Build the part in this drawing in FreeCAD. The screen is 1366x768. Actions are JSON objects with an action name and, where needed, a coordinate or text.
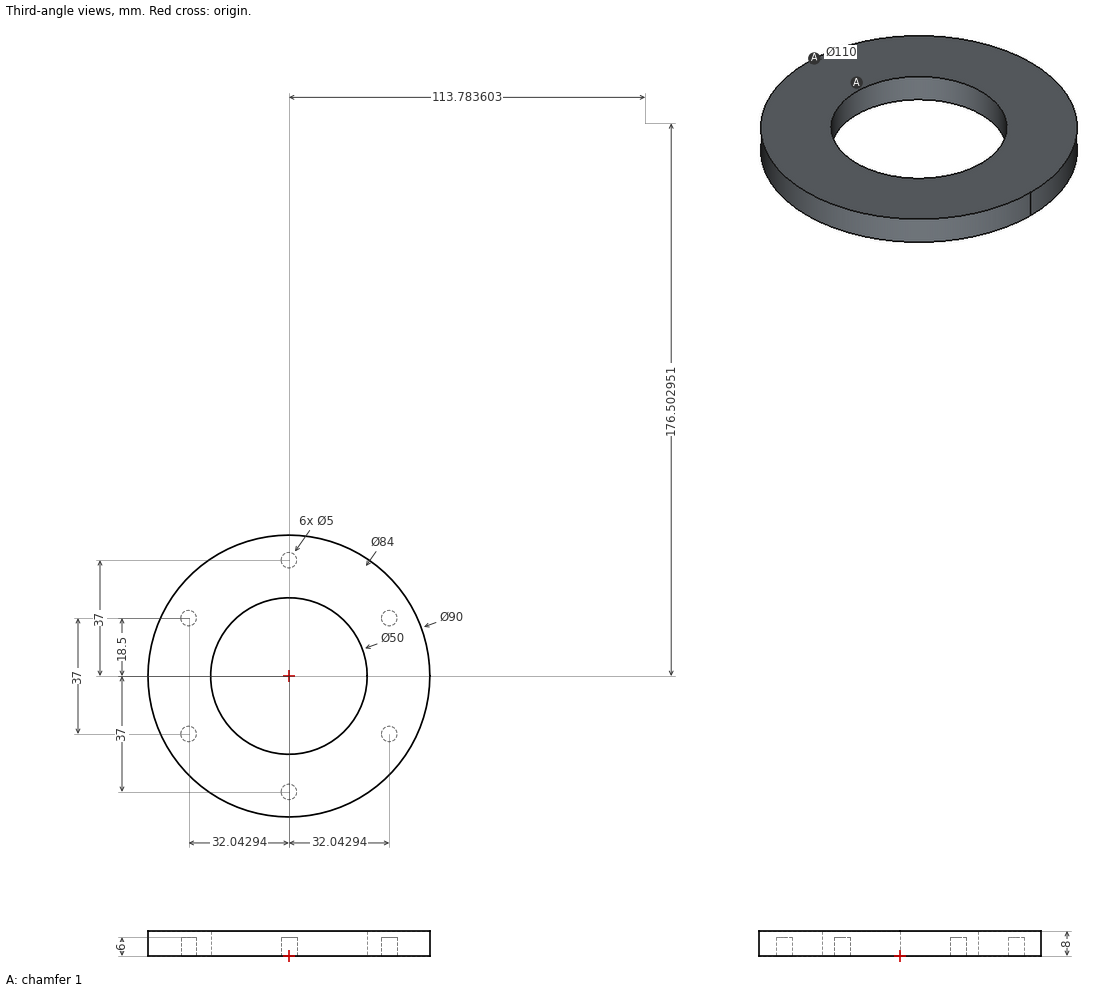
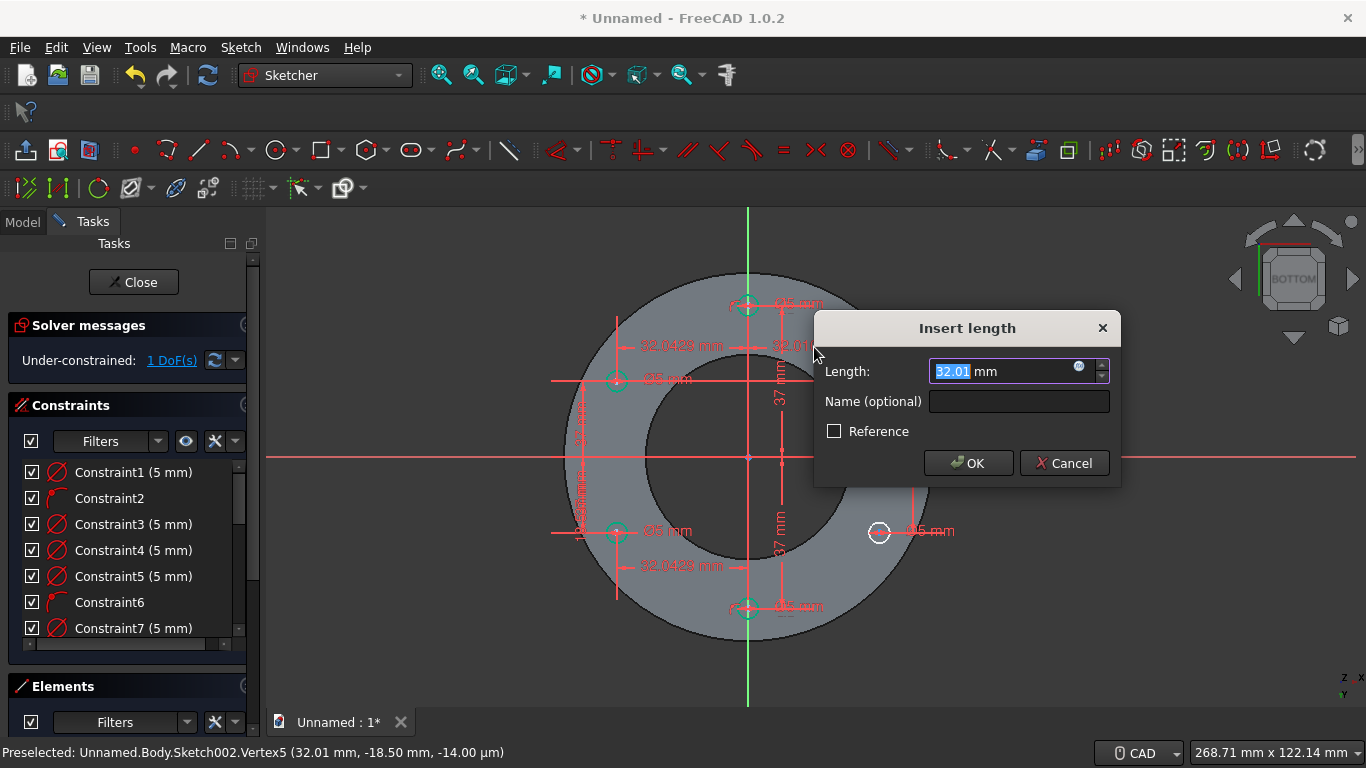
{"action": "type", "text": "32.04294"}
{"action": "key", "text": "Return"}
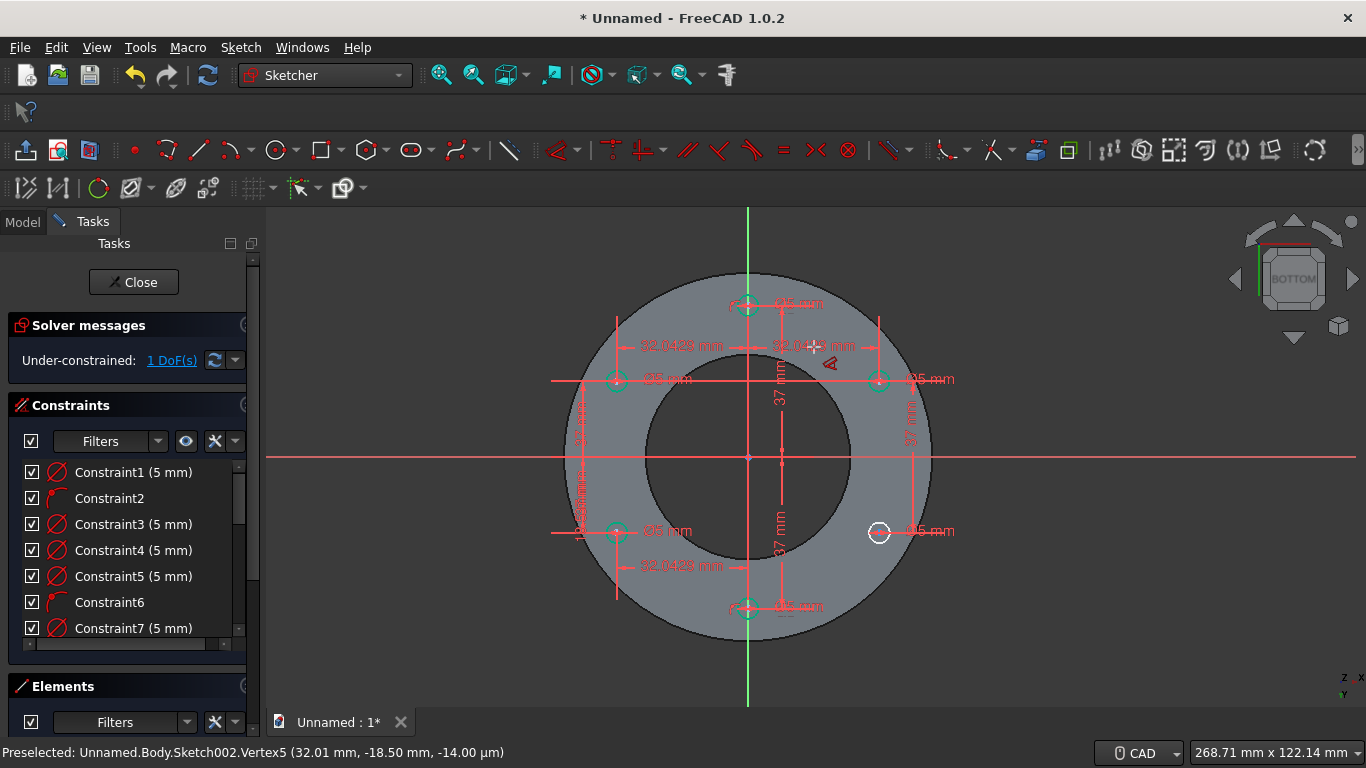
{"action": "left_click", "coordinate": [879, 533]}
{"action": "left_click", "coordinate": [814, 567]}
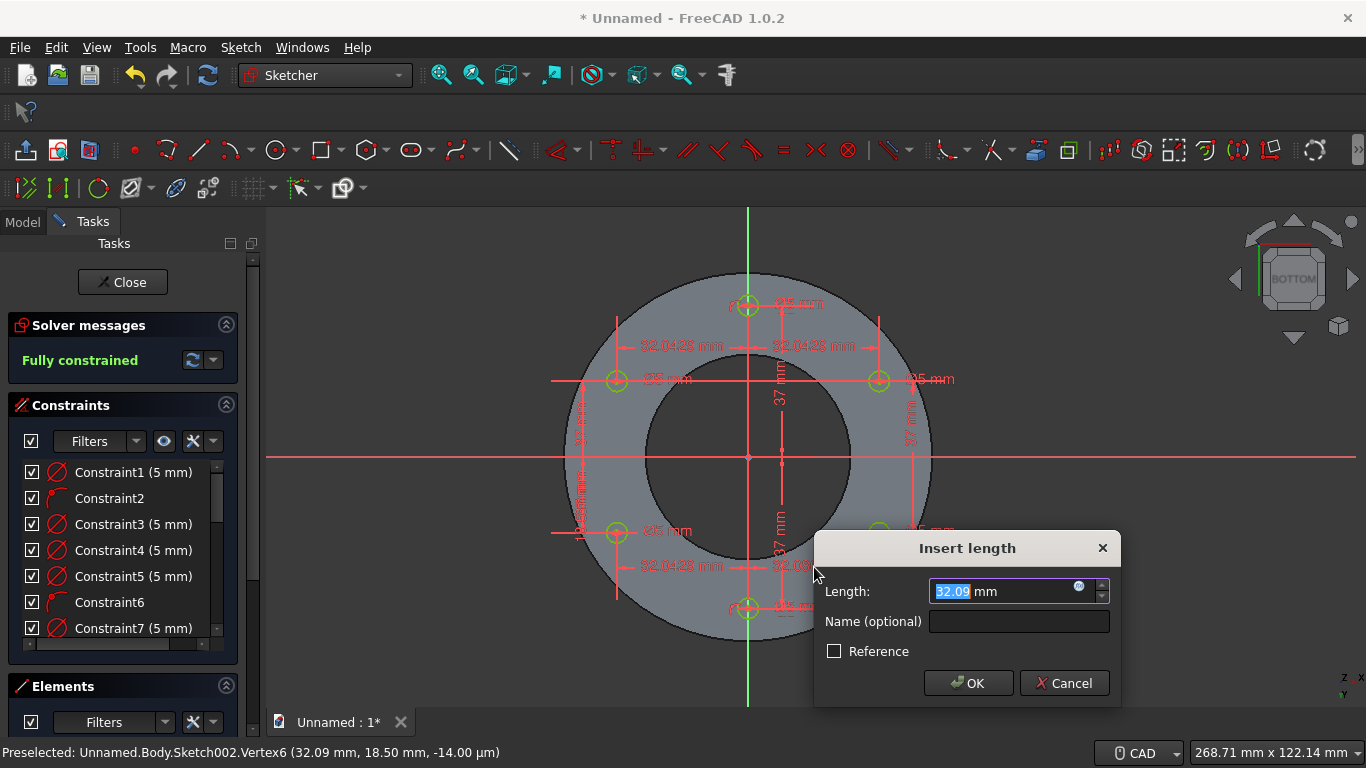
{"action": "type", "text": "32.04294"}
{"action": "key", "text": "Return"}
{"action": "key", "text": "Escape"}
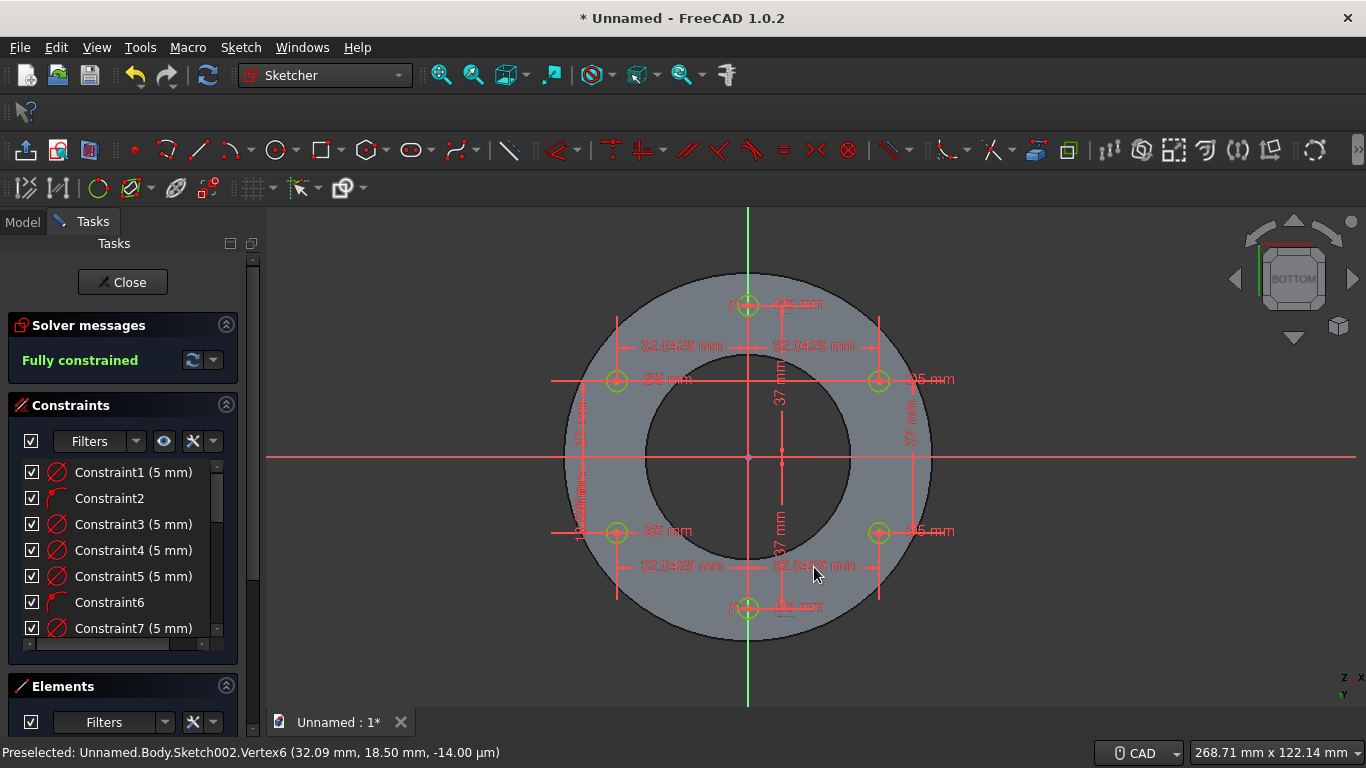
{"action": "left_click", "coordinate": [123, 282]}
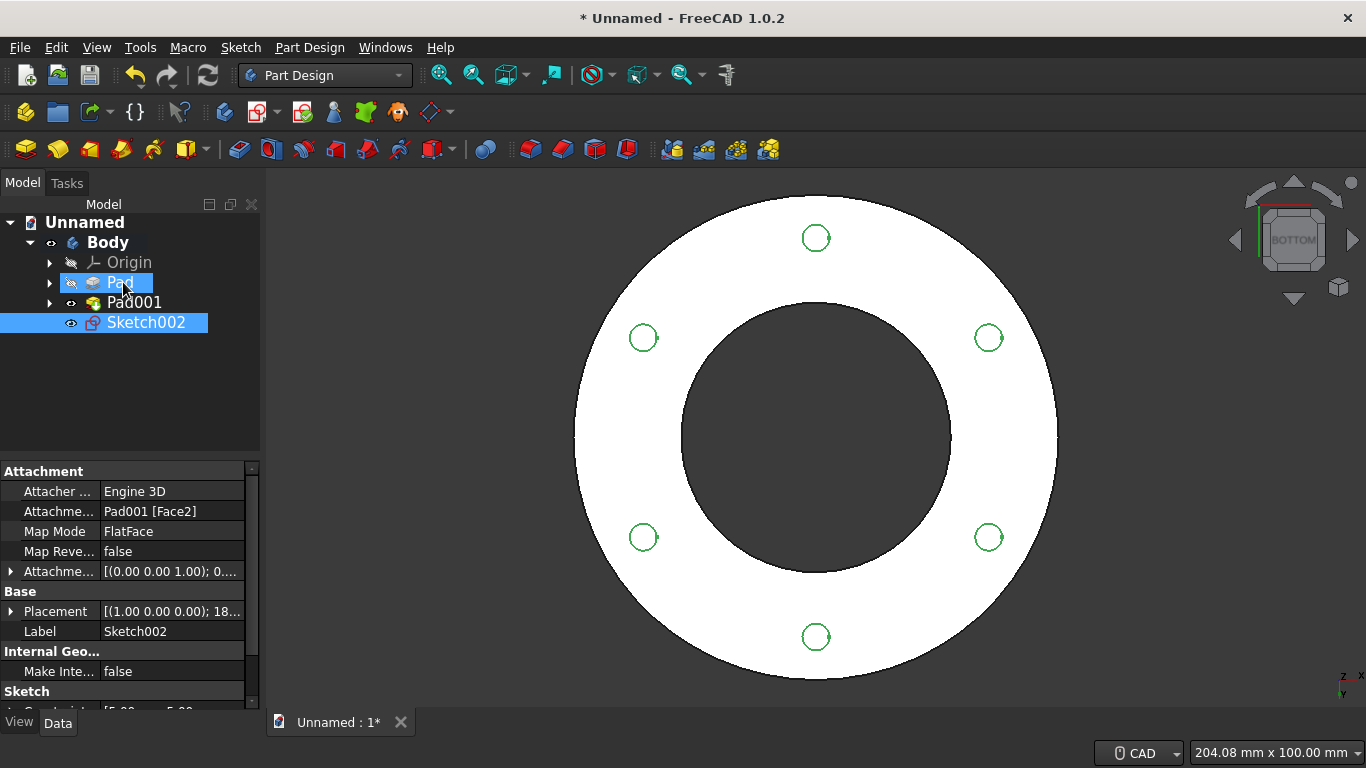
{"action": "left_click", "coordinate": [240, 150]}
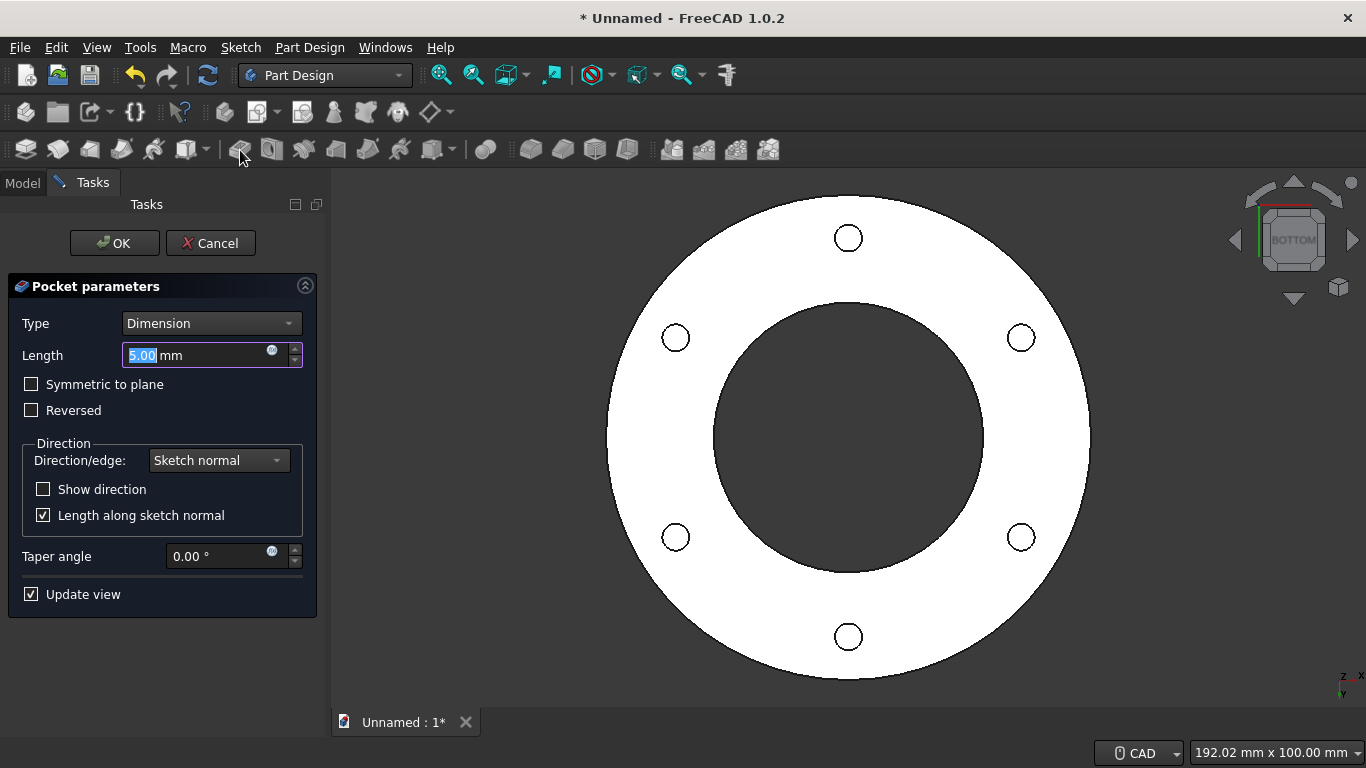
{"action": "type", "text": "6"}
{"action": "key", "text": "Tab"}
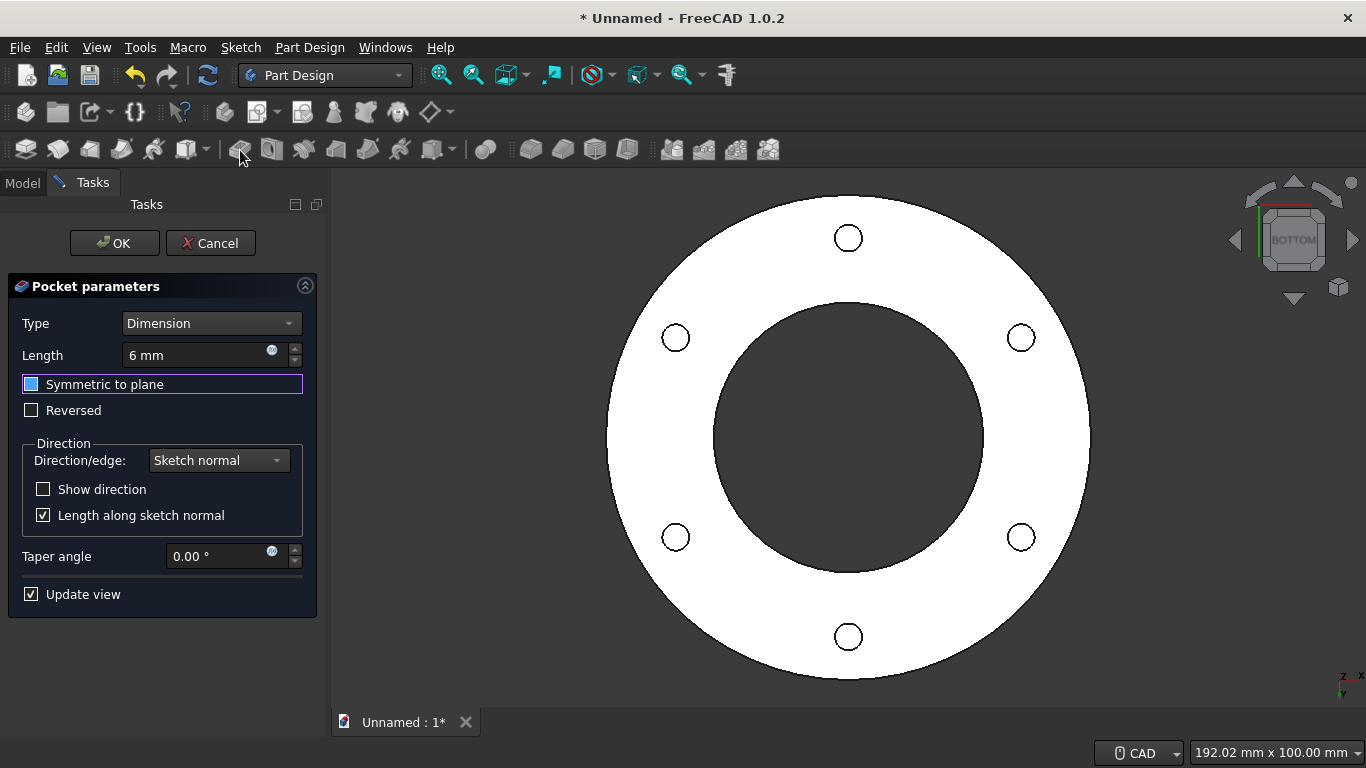
{"action": "left_click", "coordinate": [115, 243]}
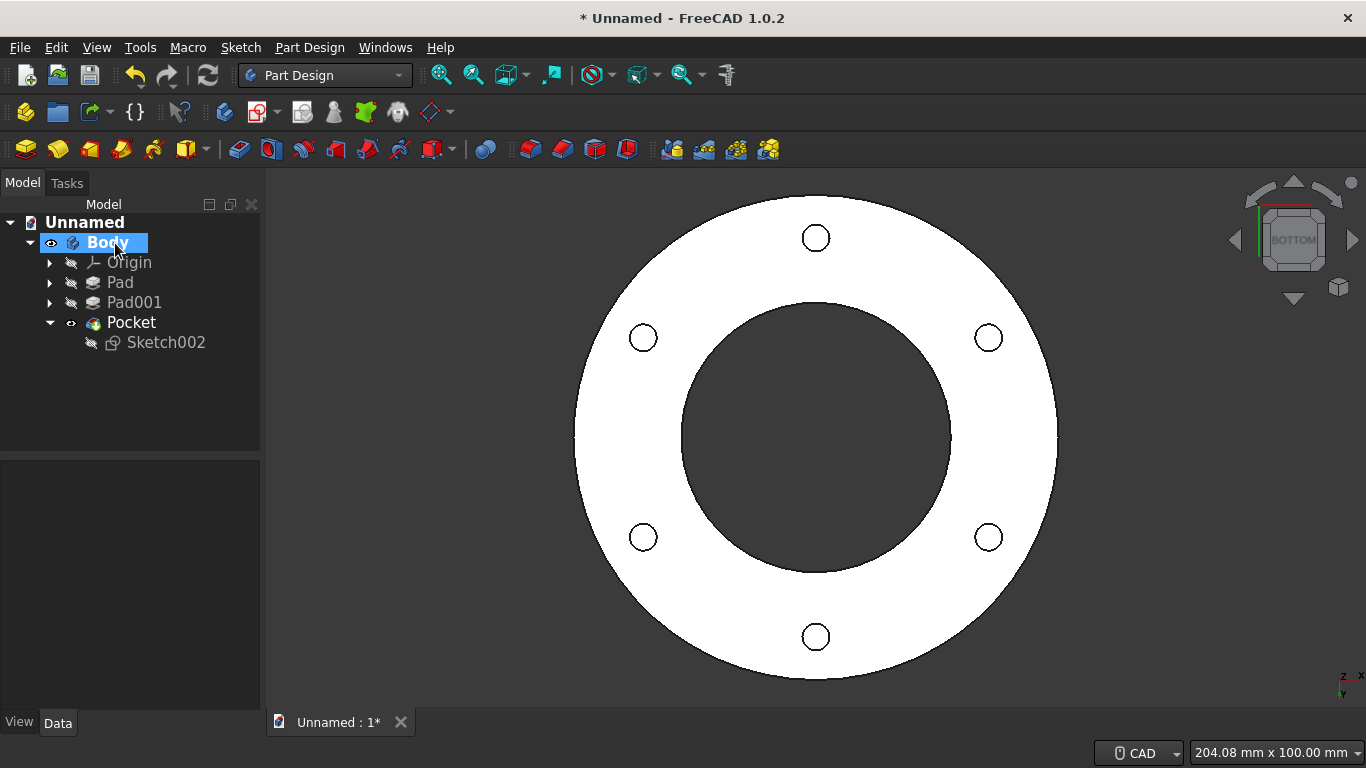
{"action": "key", "text": "0"}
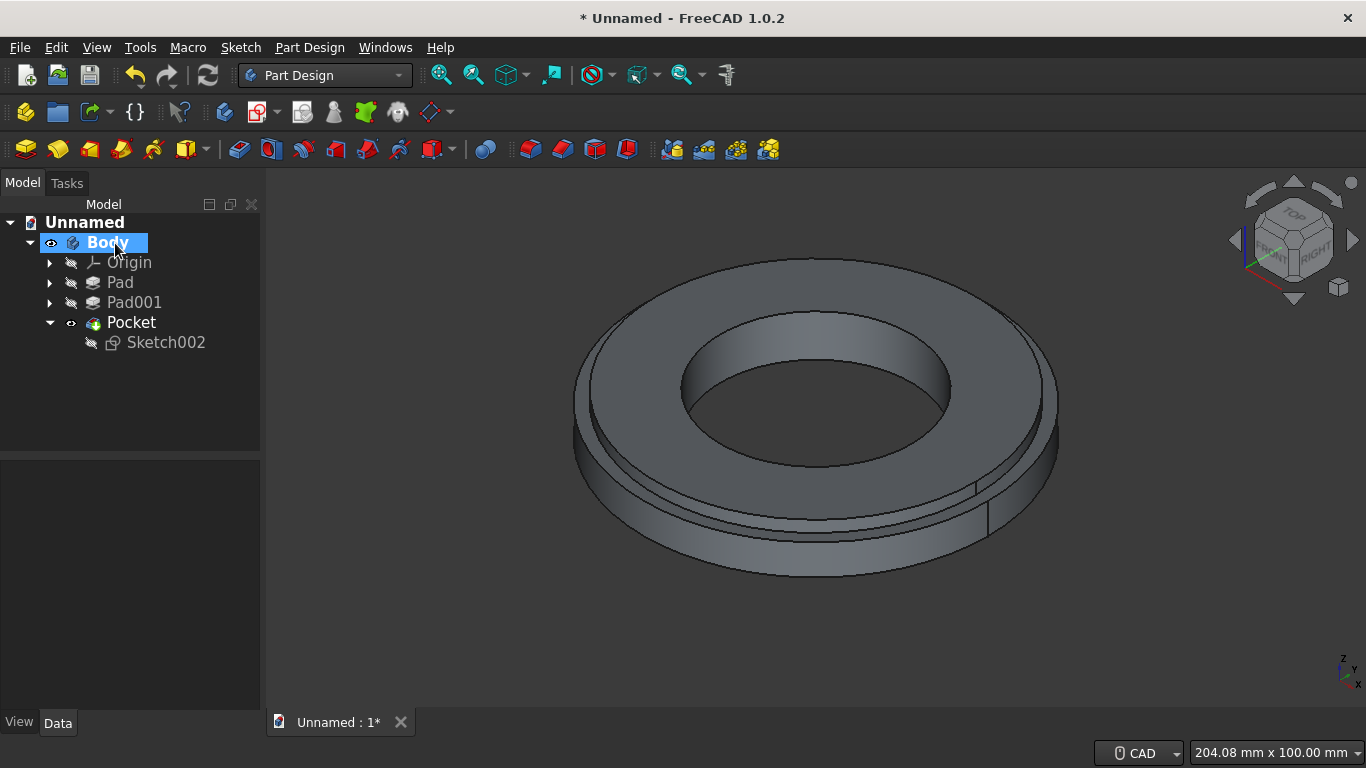
{"action": "left_click", "coordinate": [614, 447]}